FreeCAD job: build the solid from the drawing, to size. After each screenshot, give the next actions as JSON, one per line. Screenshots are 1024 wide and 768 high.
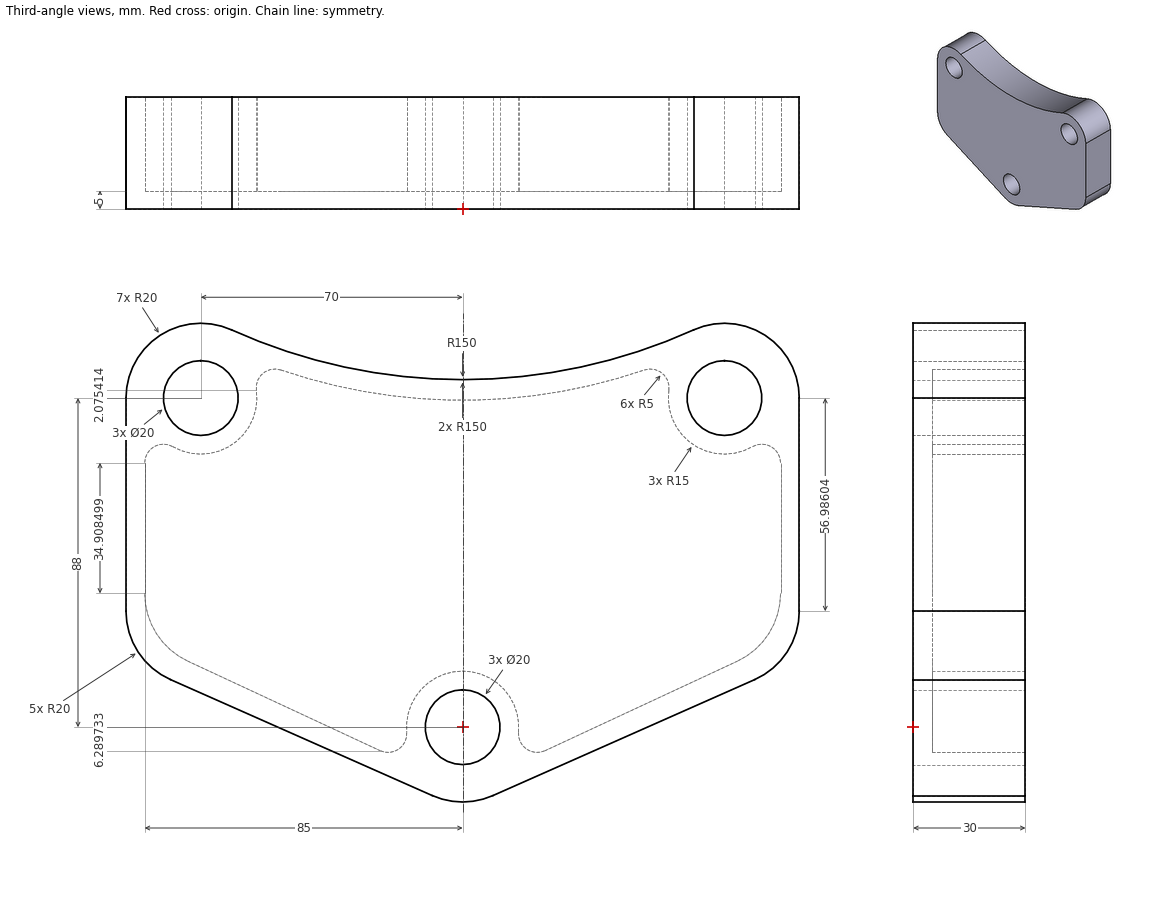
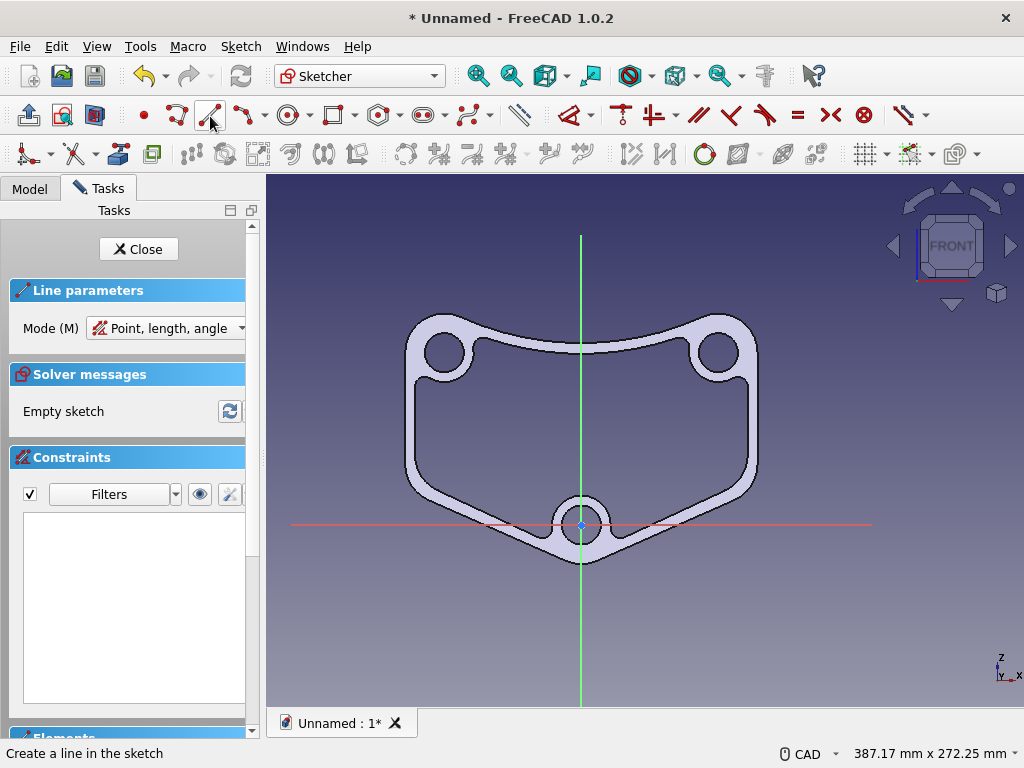
{"action": "left_click", "coordinate": [405, 353]}
{"action": "left_click", "coordinate": [405, 464]}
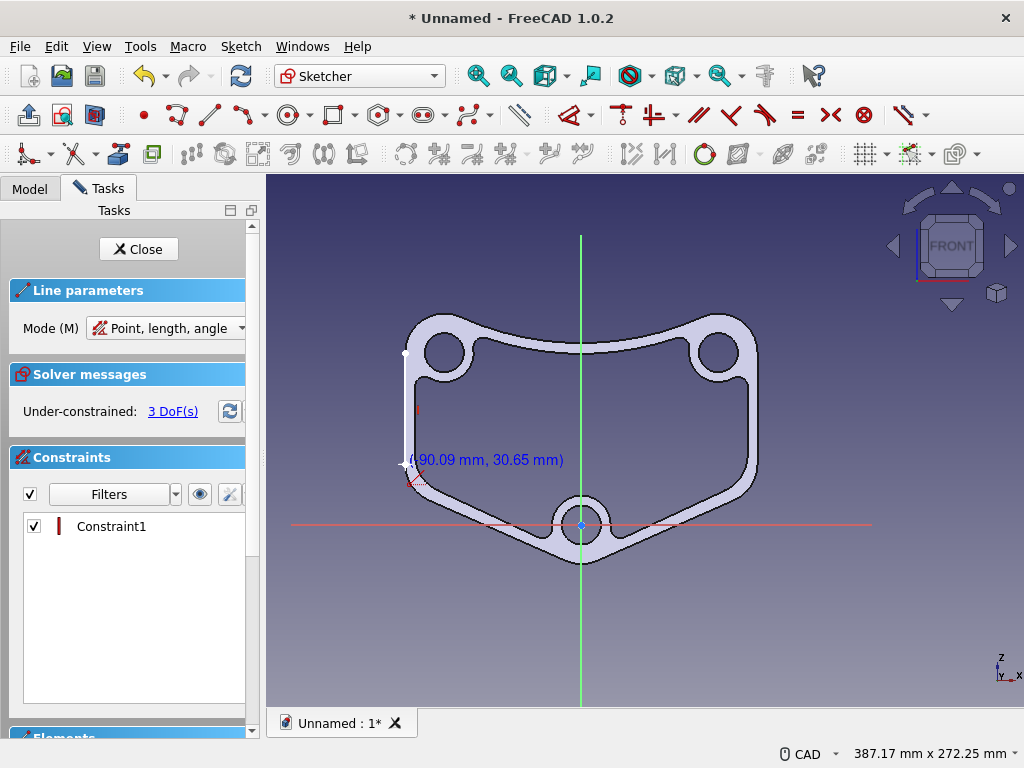
{"action": "left_click", "coordinate": [428, 500]}
{"action": "left_click", "coordinate": [566, 561]}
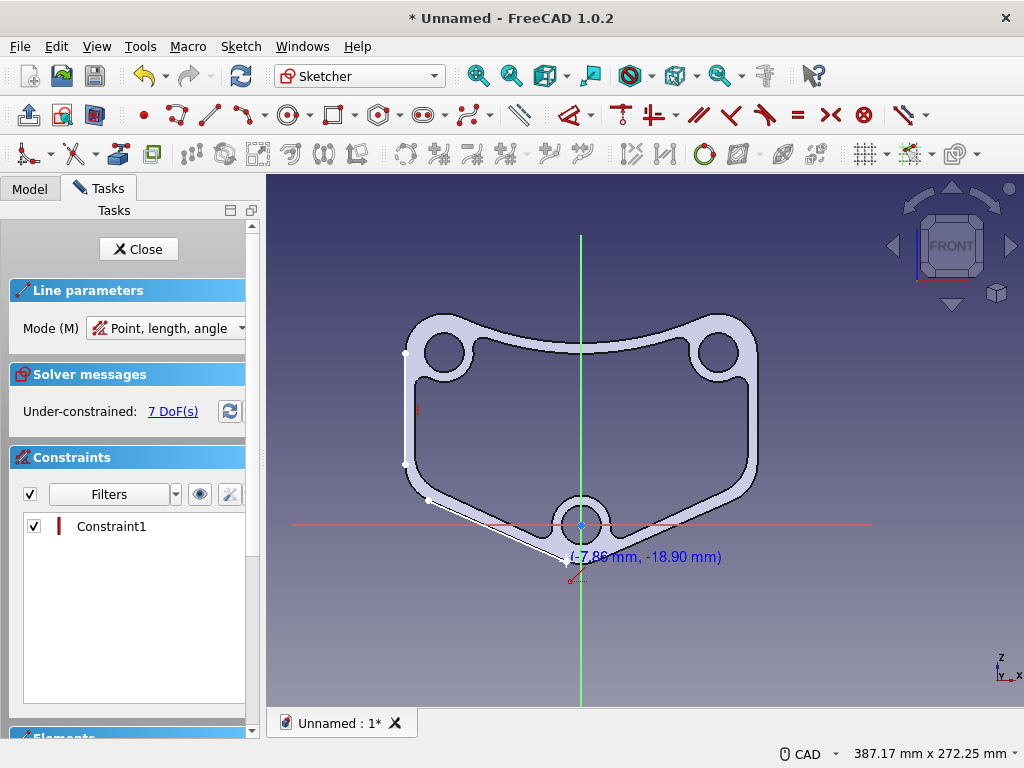
{"action": "left_click", "coordinate": [597, 561]}
{"action": "left_click", "coordinate": [734, 500]}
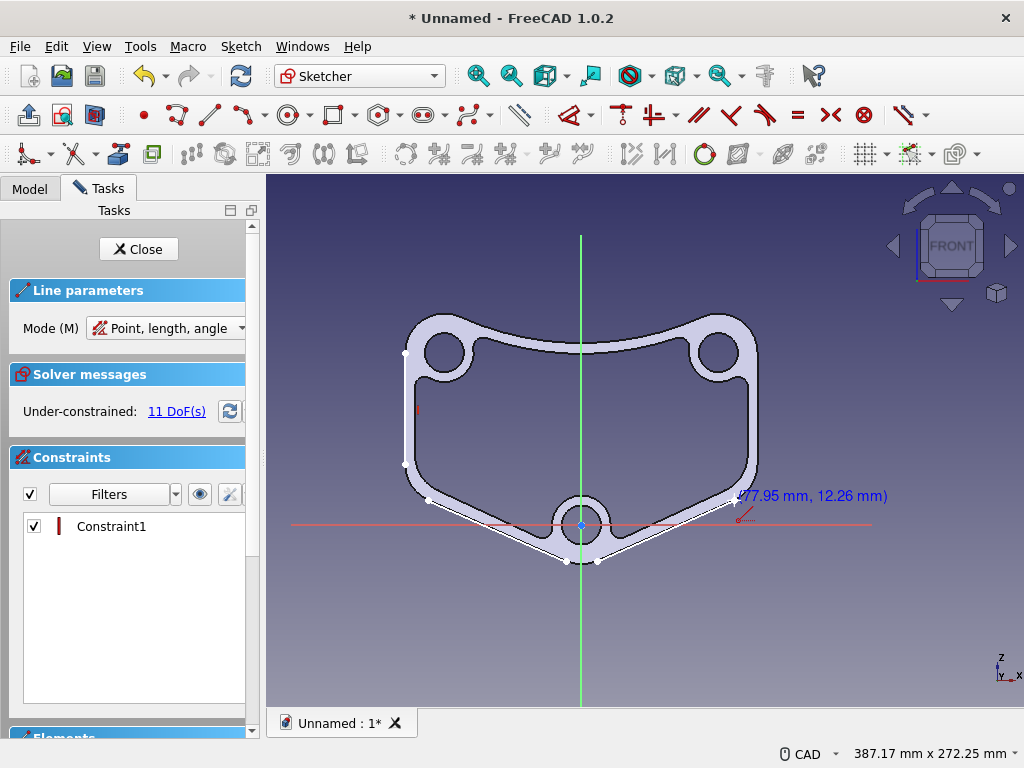
{"action": "left_click", "coordinate": [758, 464]}
{"action": "left_click", "coordinate": [758, 353]}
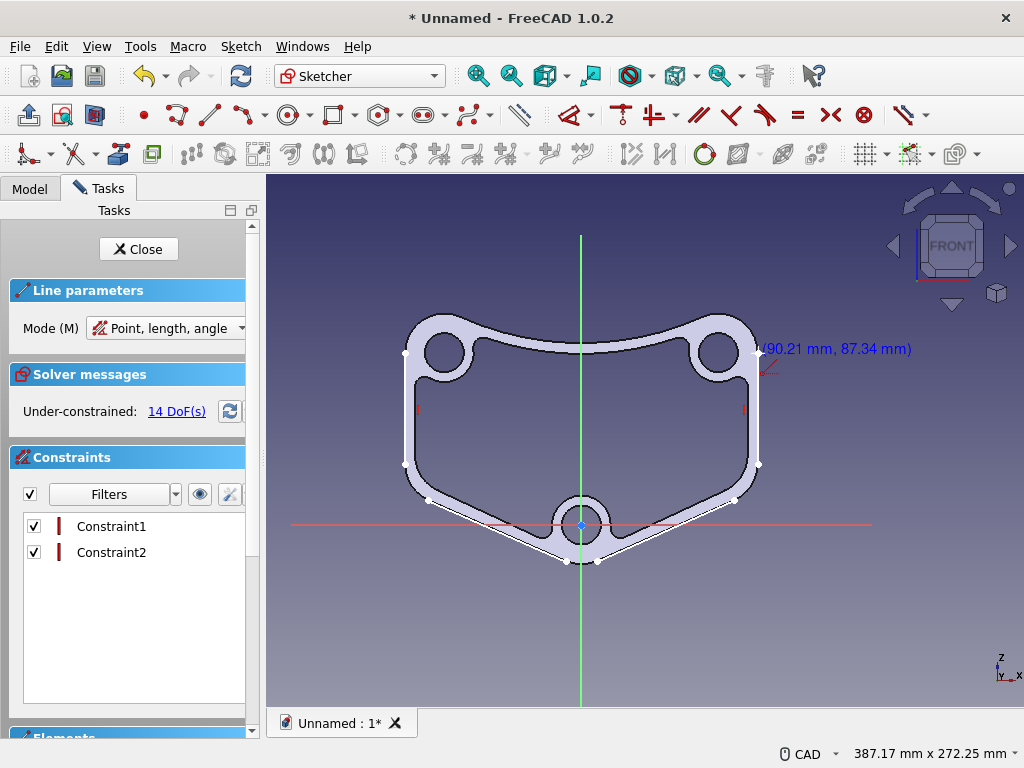
{"action": "left_click", "coordinate": [242, 116]}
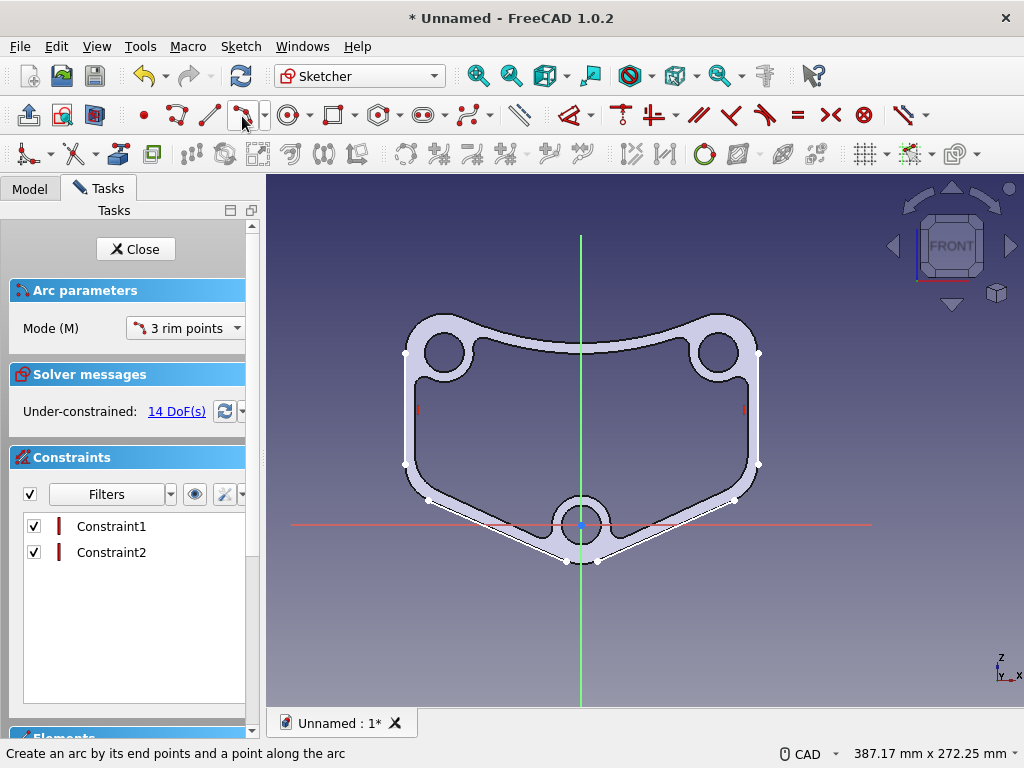
{"action": "left_click", "coordinate": [405, 465]}
{"action": "left_click", "coordinate": [428, 501]}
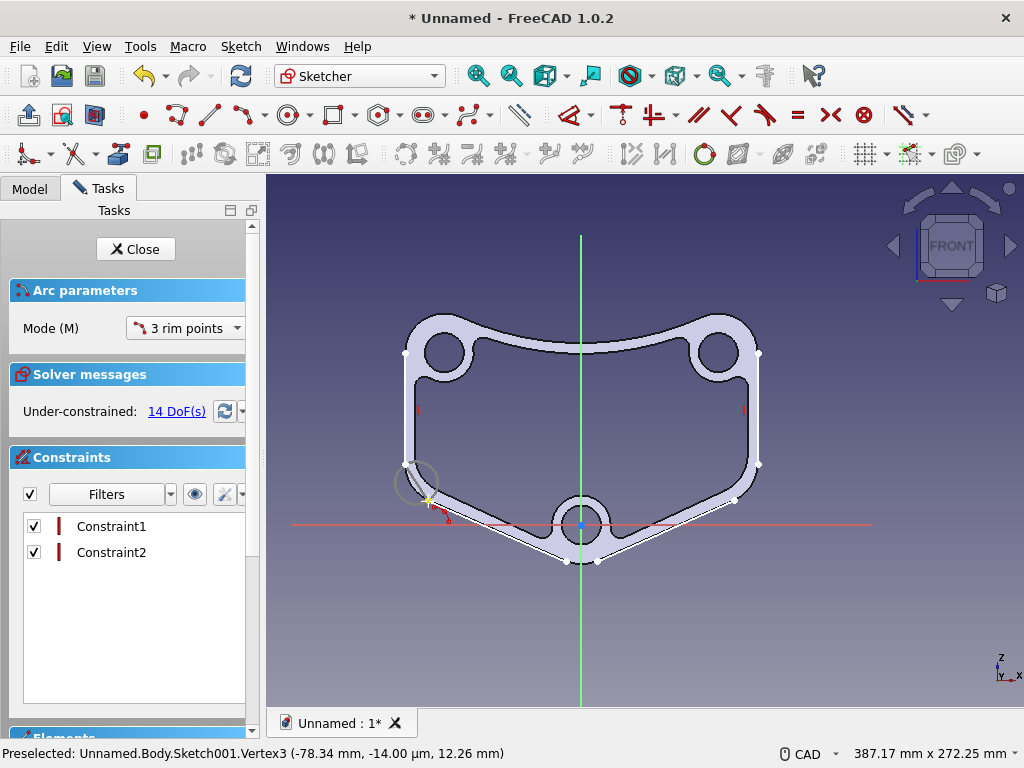
{"action": "scroll", "coordinate": [412, 486], "scroll_direction": "up", "scroll_amount": 5}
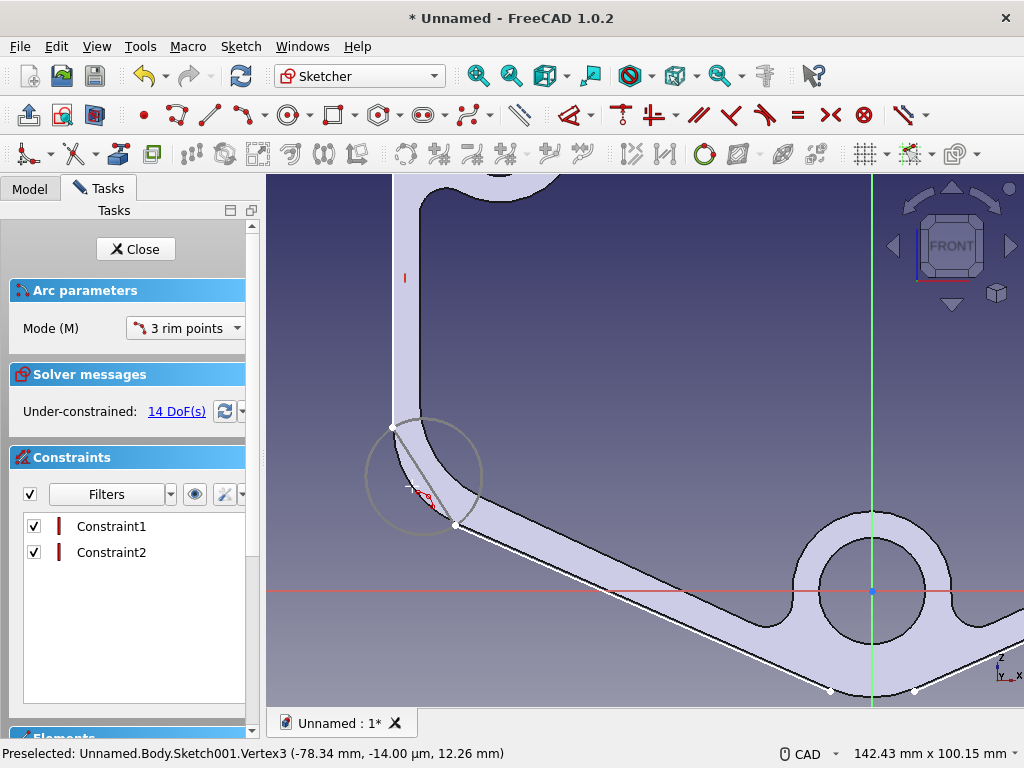
{"action": "left_click", "coordinate": [410, 484]}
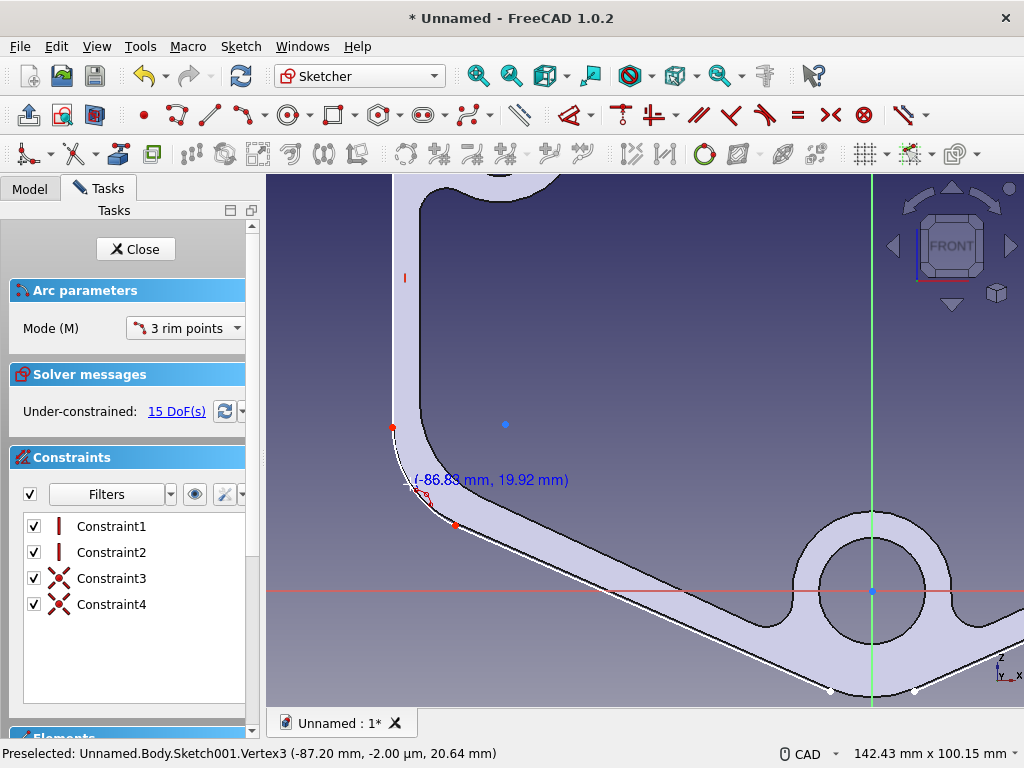
{"action": "scroll", "coordinate": [335, 505], "scroll_direction": "down", "scroll_amount": 4}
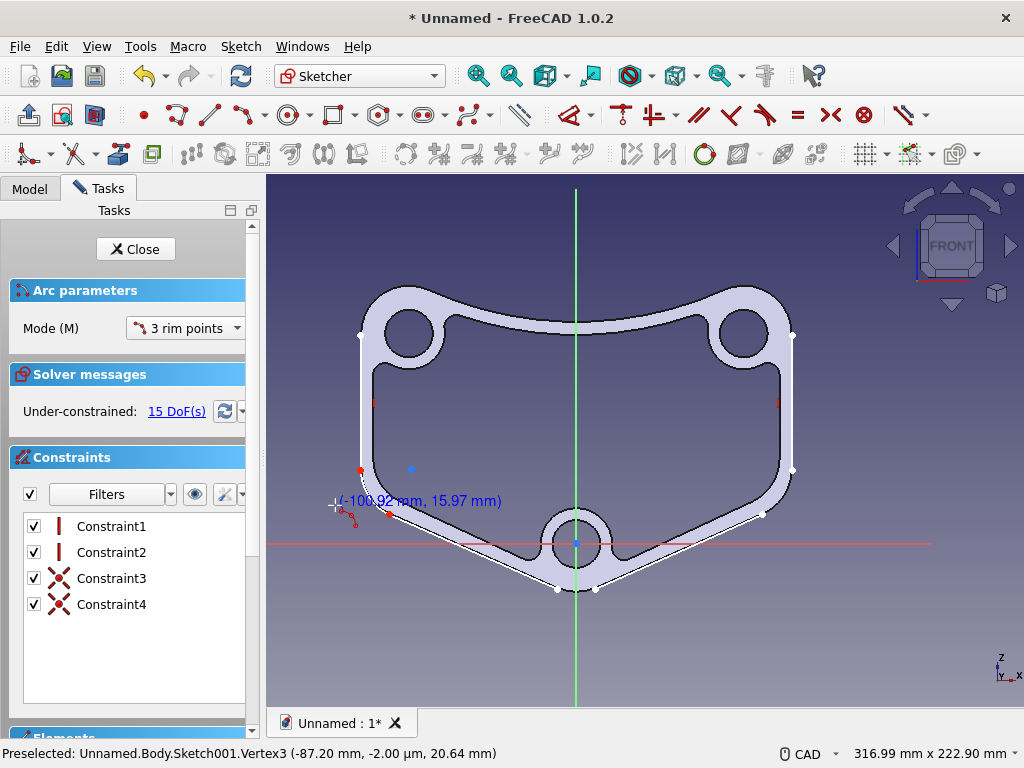
{"action": "left_click", "coordinate": [558, 589]}
{"action": "left_click", "coordinate": [595, 589]}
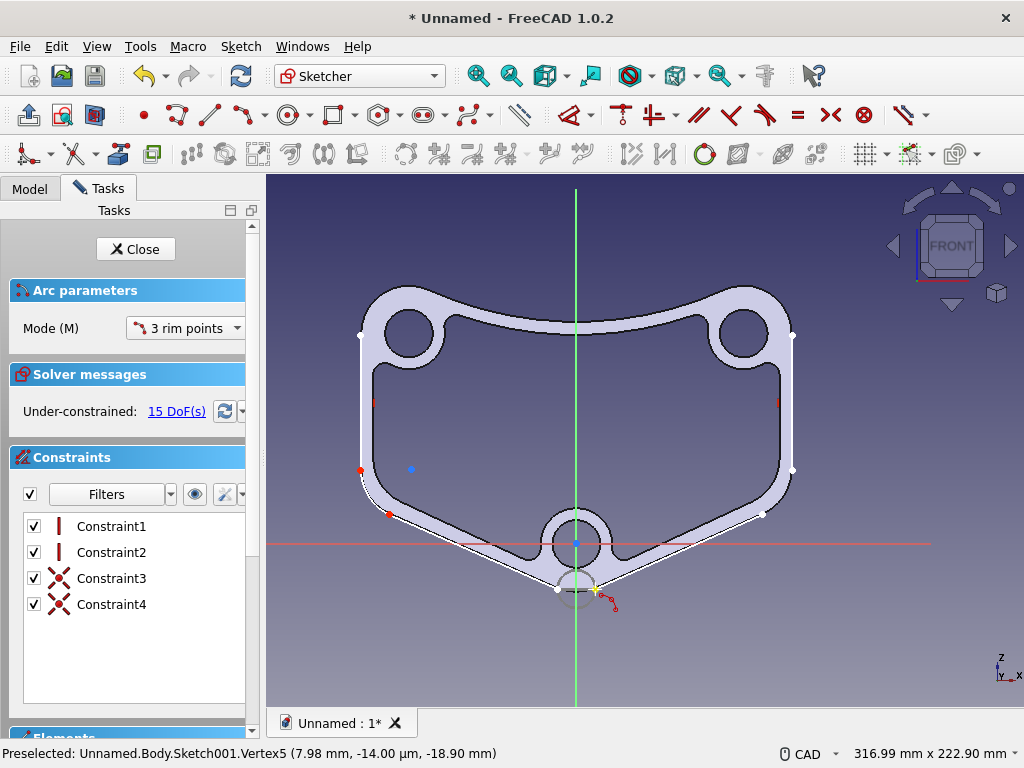
{"action": "scroll", "coordinate": [572, 592], "scroll_direction": "up", "scroll_amount": 7}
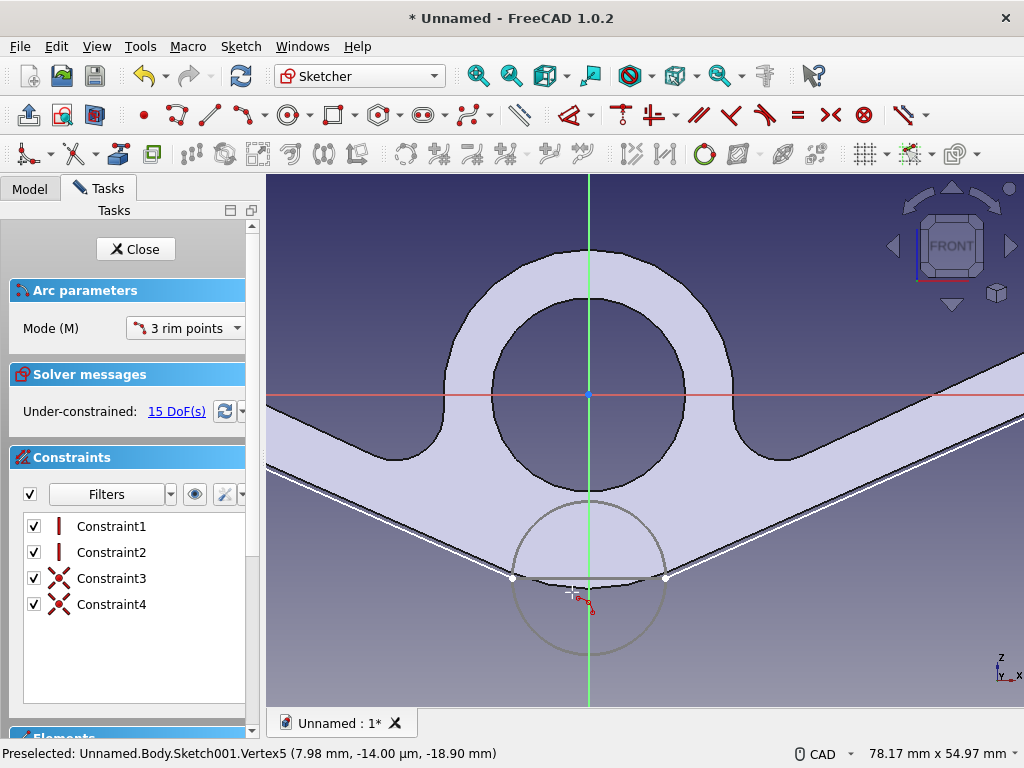
{"action": "left_click", "coordinate": [572, 588]}